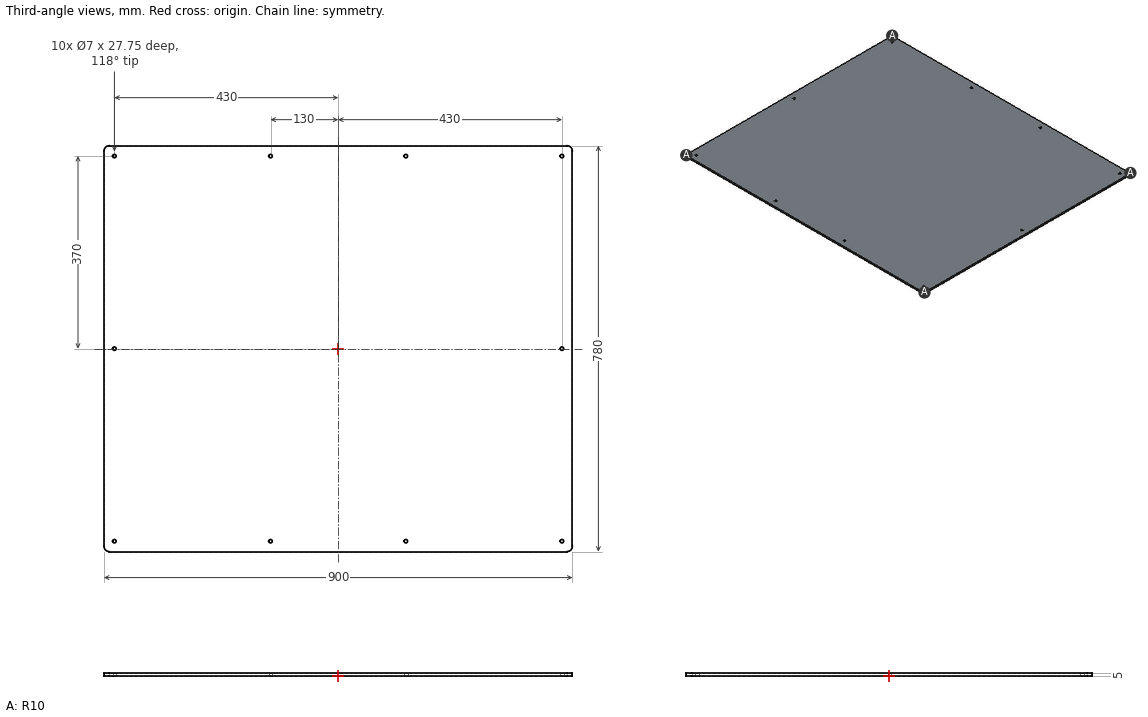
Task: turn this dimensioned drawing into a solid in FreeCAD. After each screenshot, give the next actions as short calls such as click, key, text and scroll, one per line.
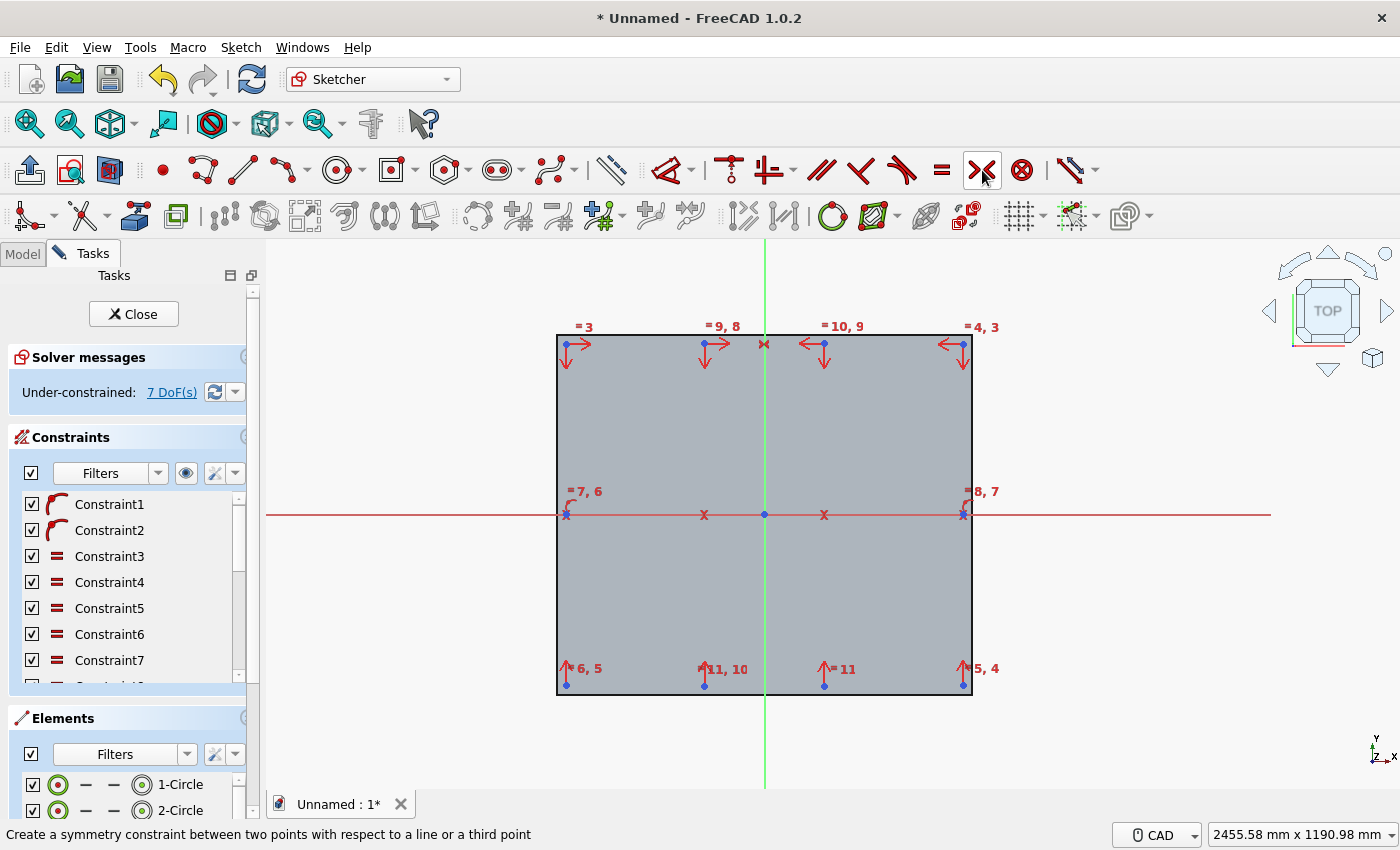
click(666, 170)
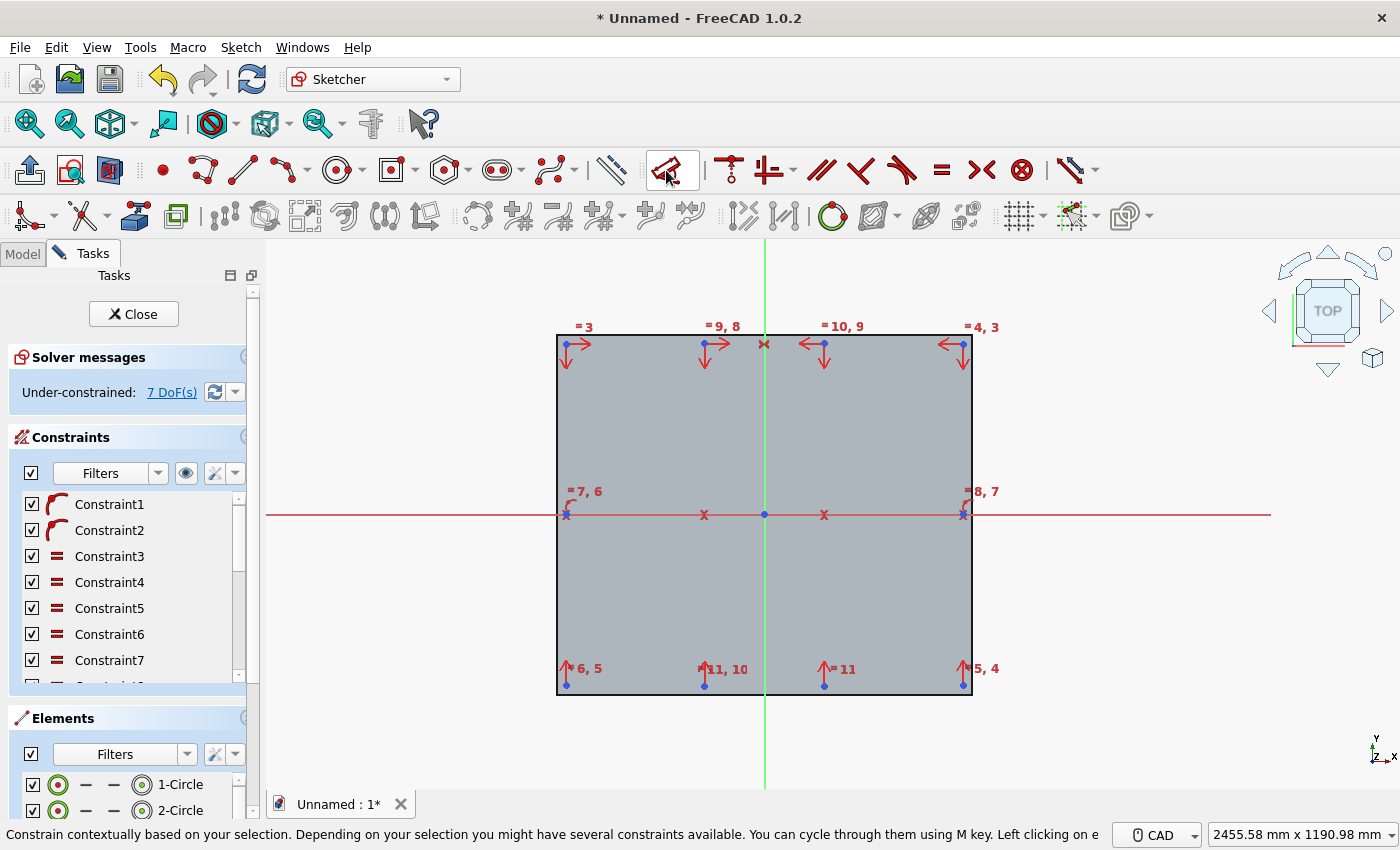
scroll(568, 343, up, 13)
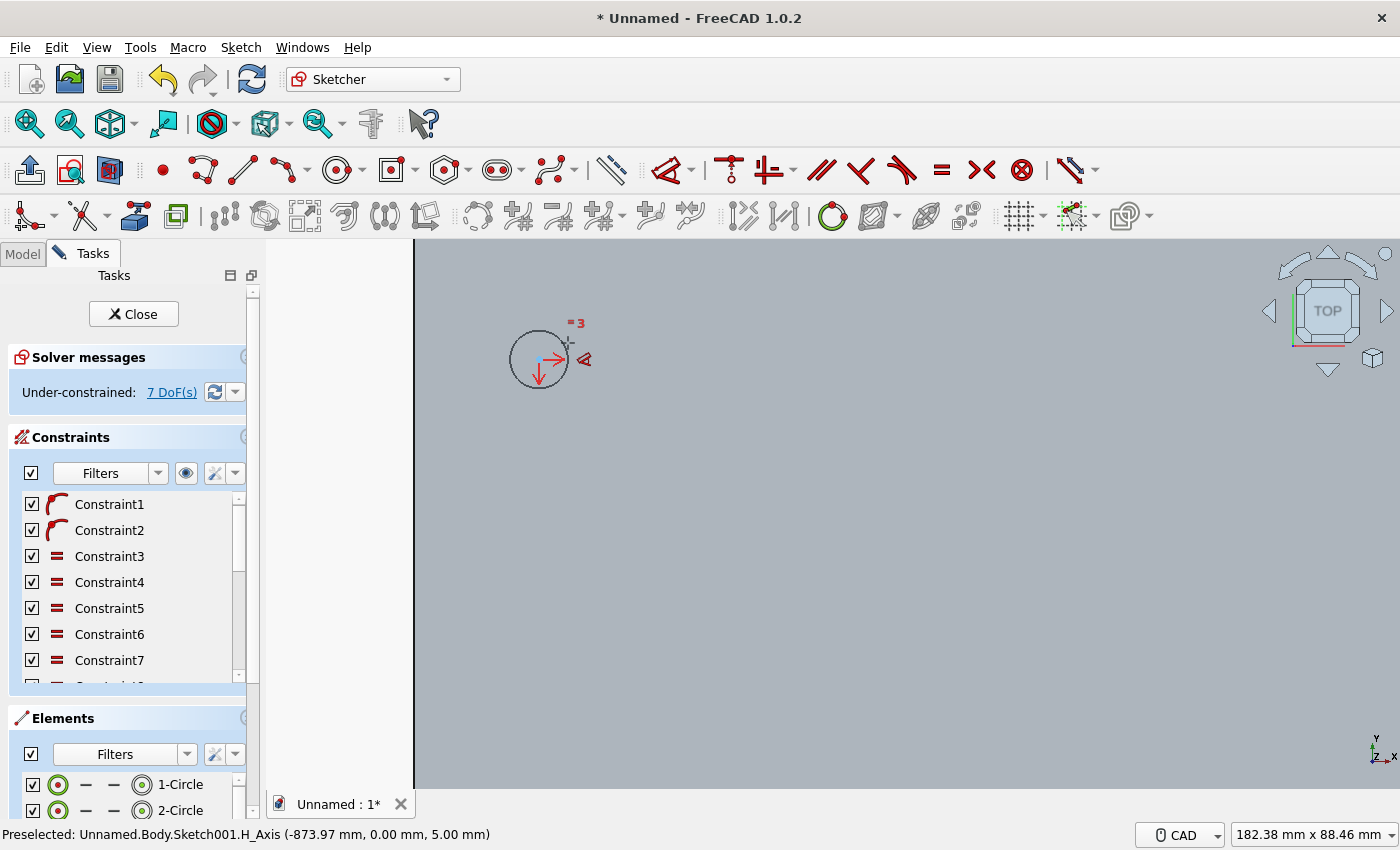
click(559, 339)
click(581, 316)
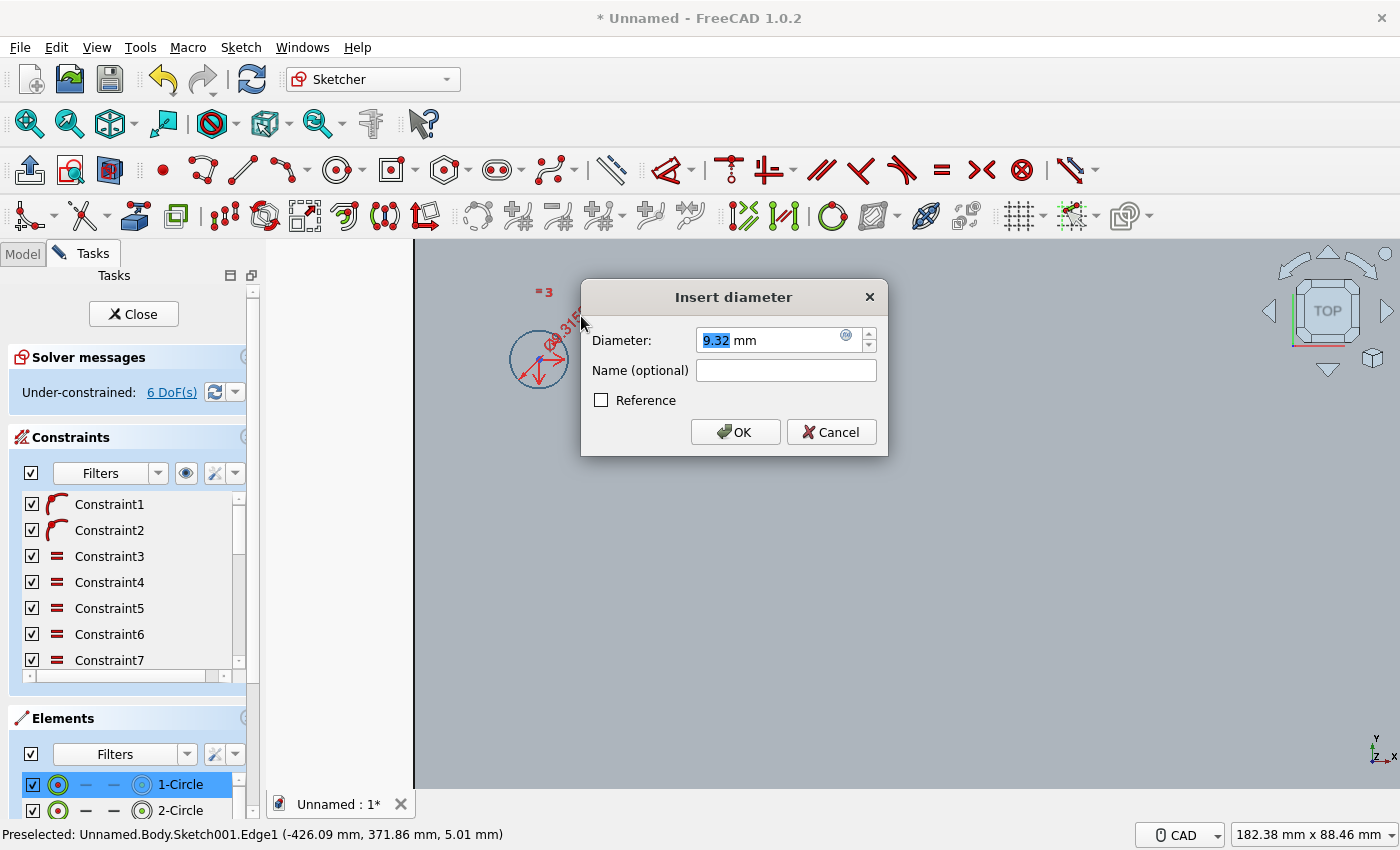
text(7)
key(Return)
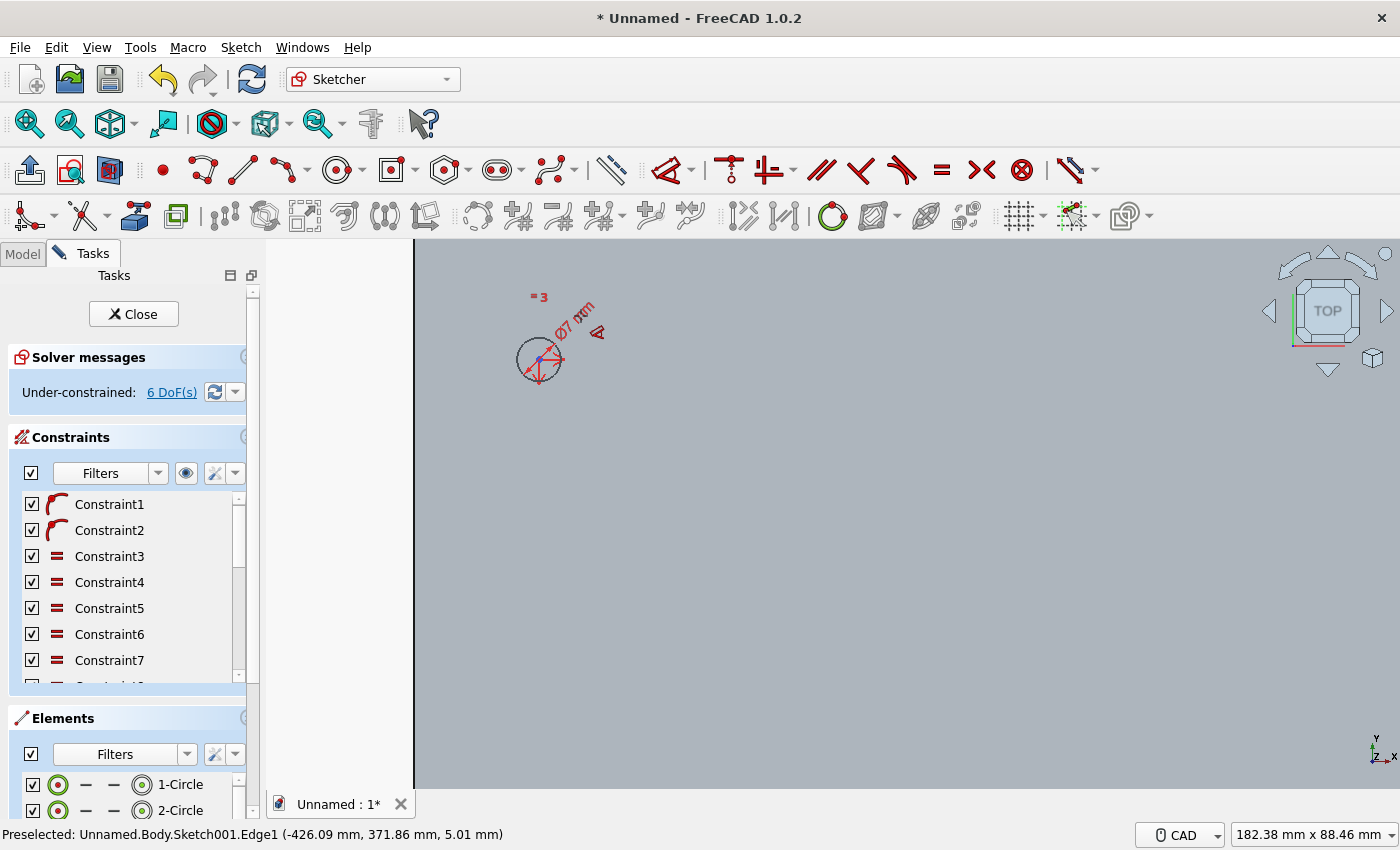
scroll(568, 342, down, 13)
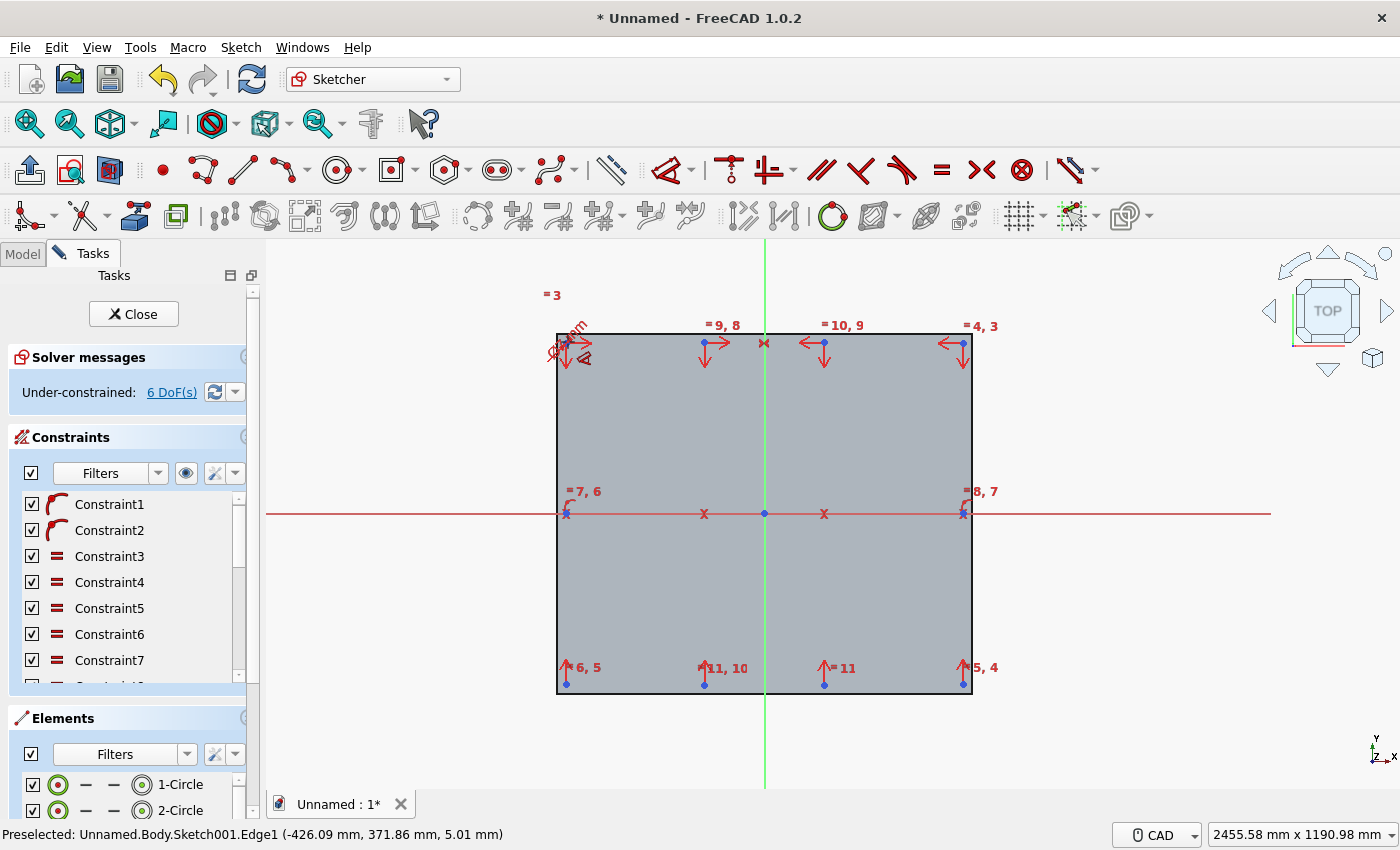
click(566, 343)
click(665, 309)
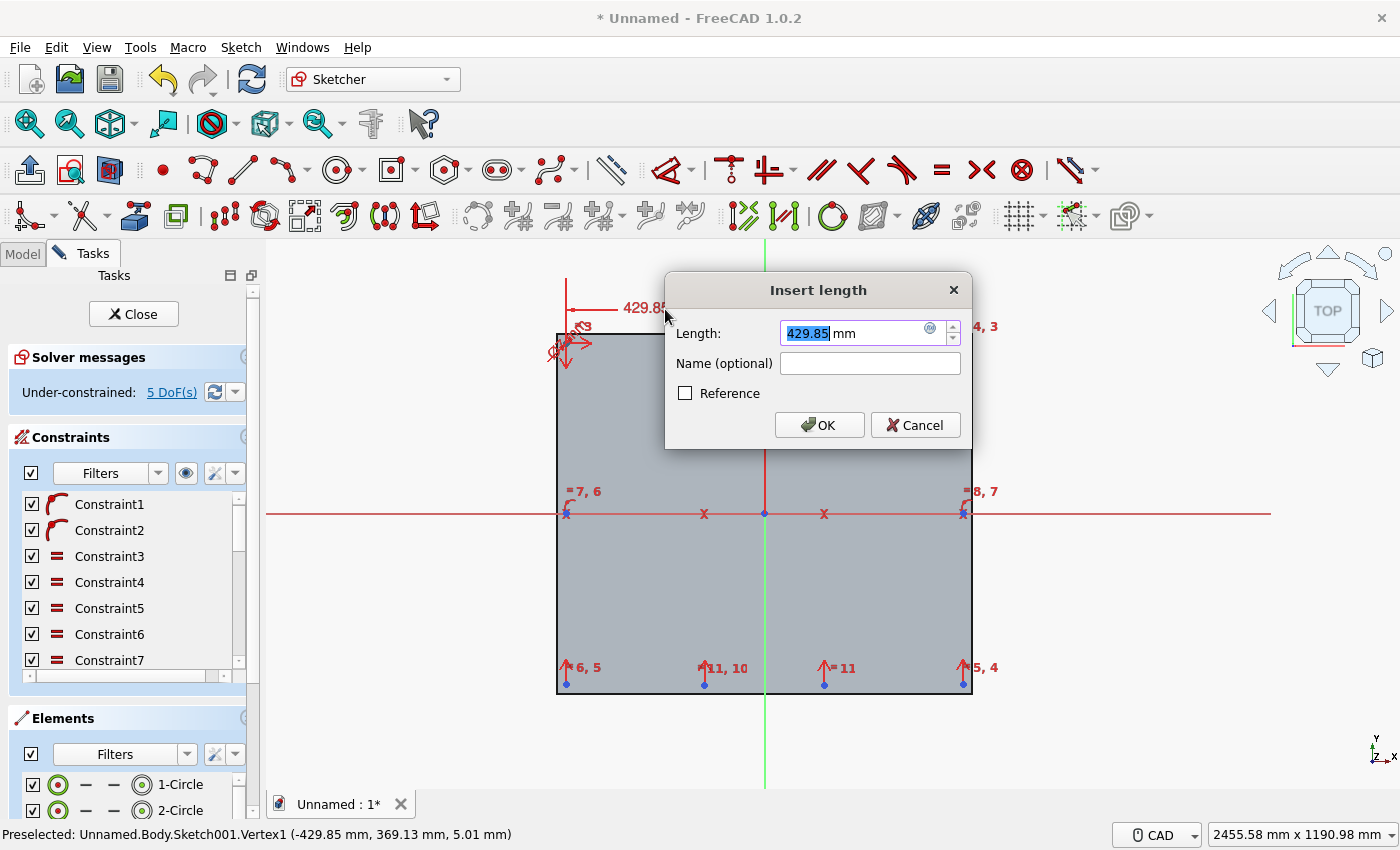
text(430)
key(Return)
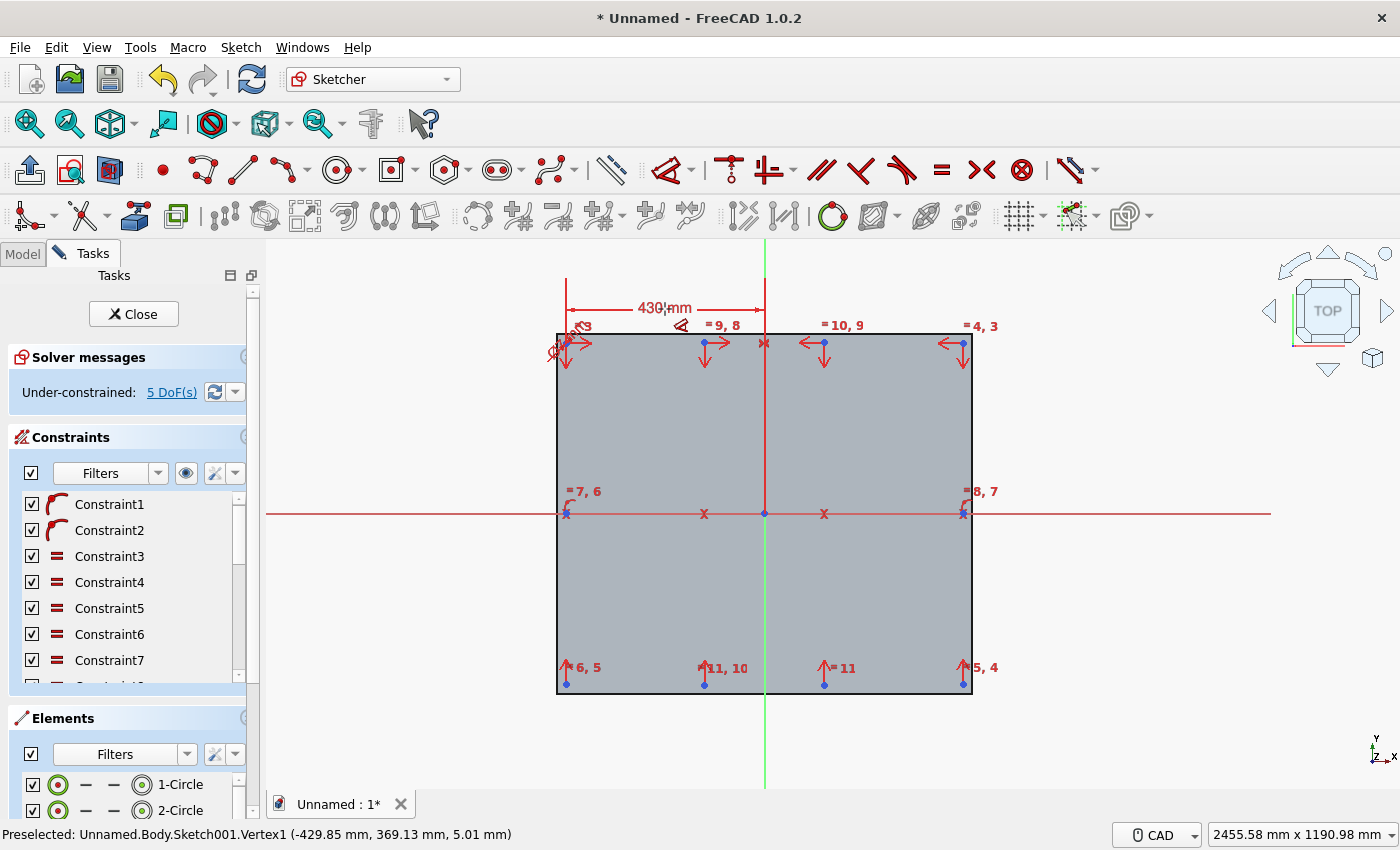
click(566, 343)
click(532, 429)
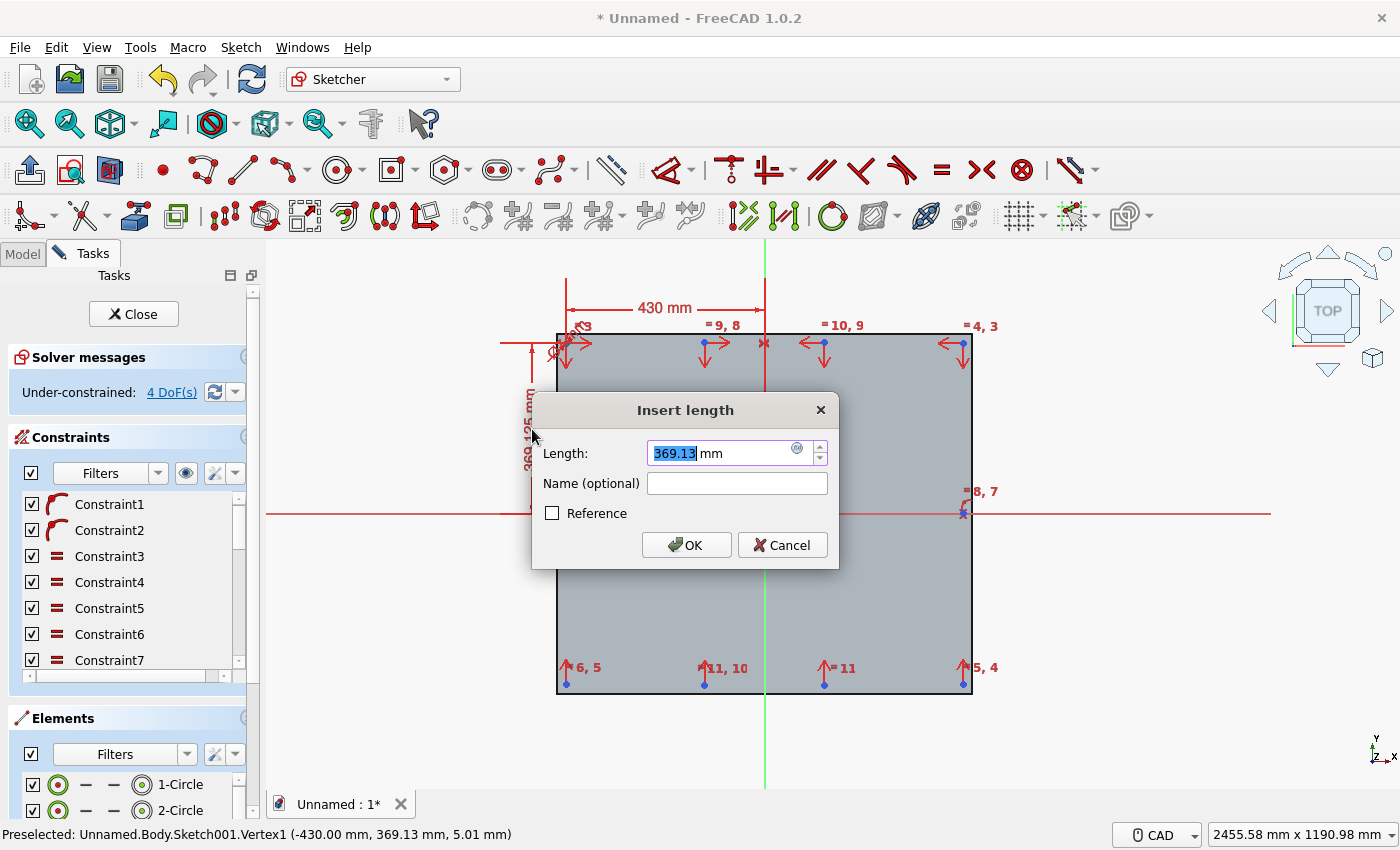
text(370)
key(Return)